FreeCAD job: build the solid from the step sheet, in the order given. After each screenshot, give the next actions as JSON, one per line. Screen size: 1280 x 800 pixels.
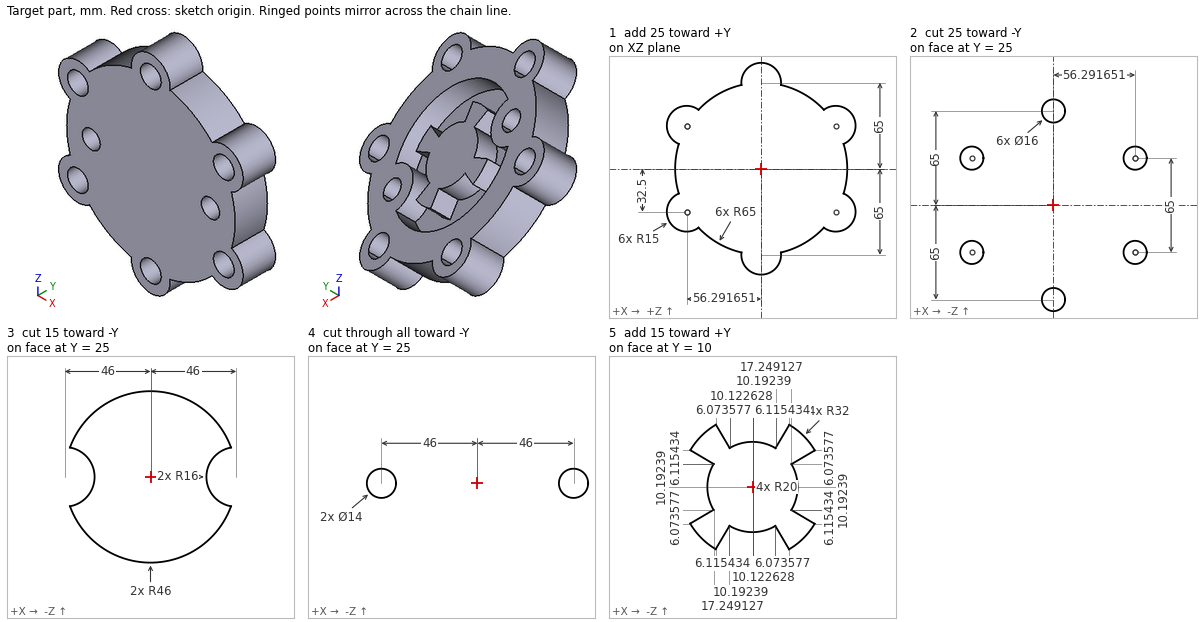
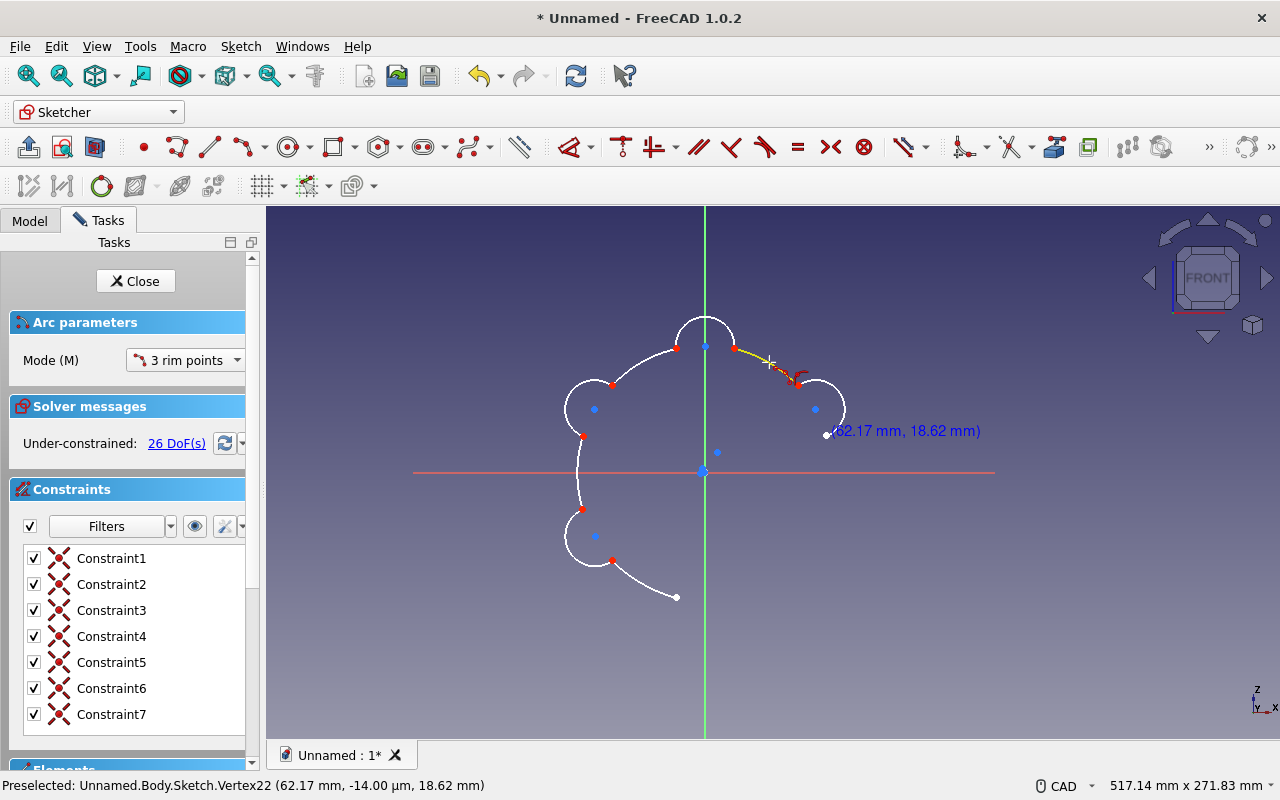
{"action": "left_click", "coordinate": [827, 509]}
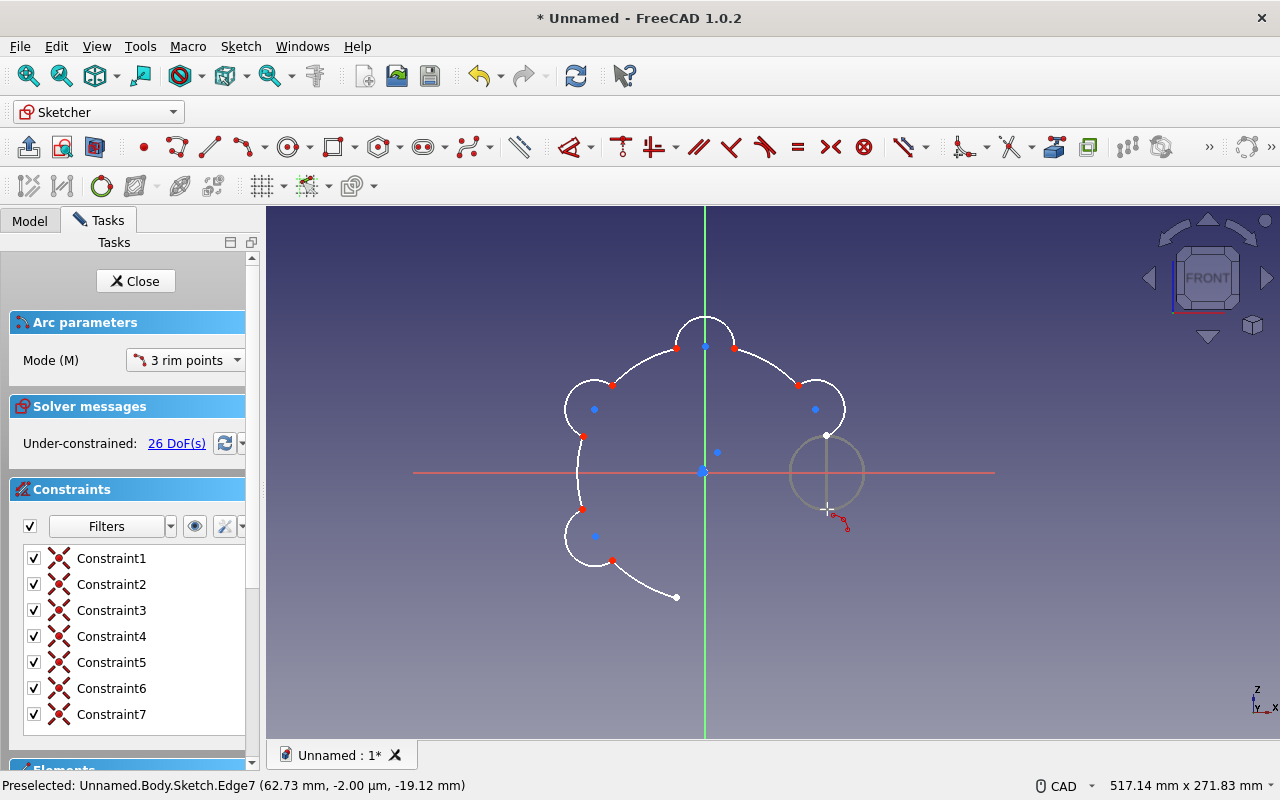
{"action": "scroll", "coordinate": [832, 480], "scroll_direction": "up", "scroll_amount": 6}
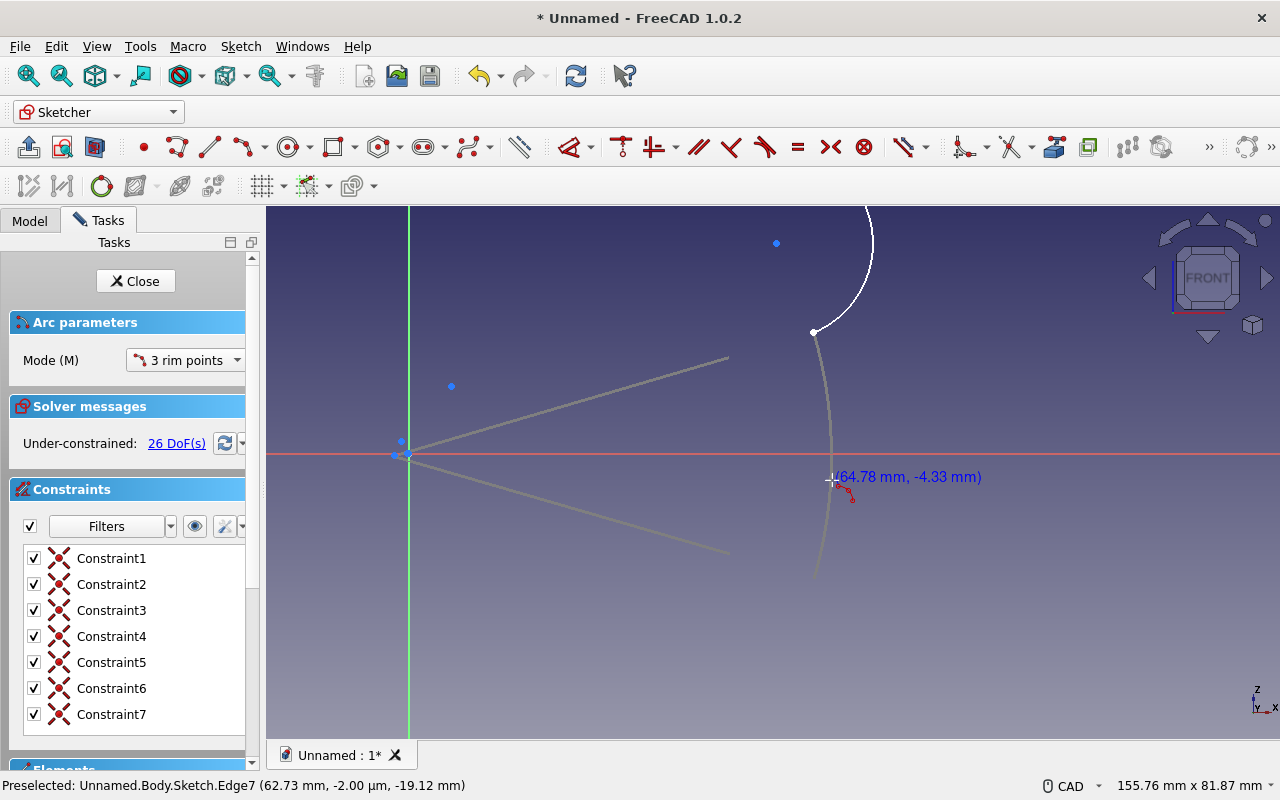
{"action": "left_click", "coordinate": [831, 479]}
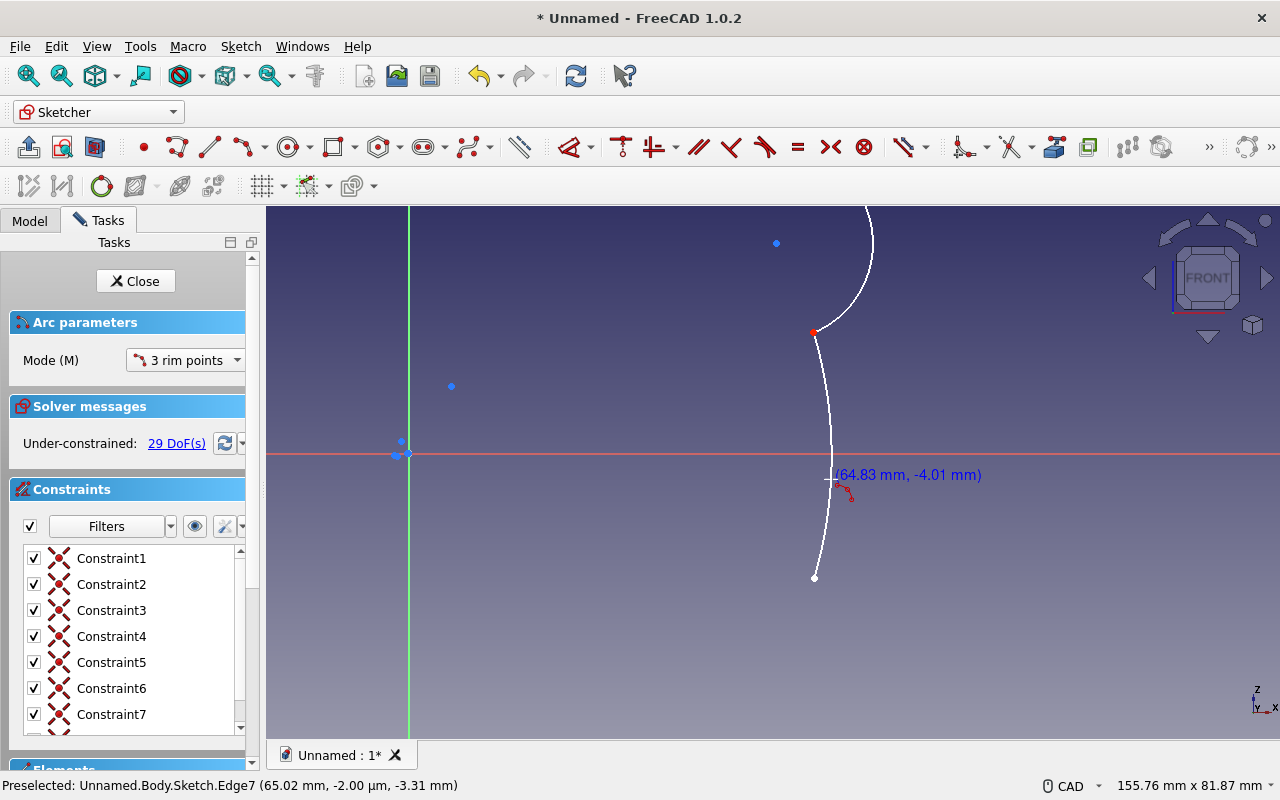
{"action": "left_click", "coordinate": [814, 578]}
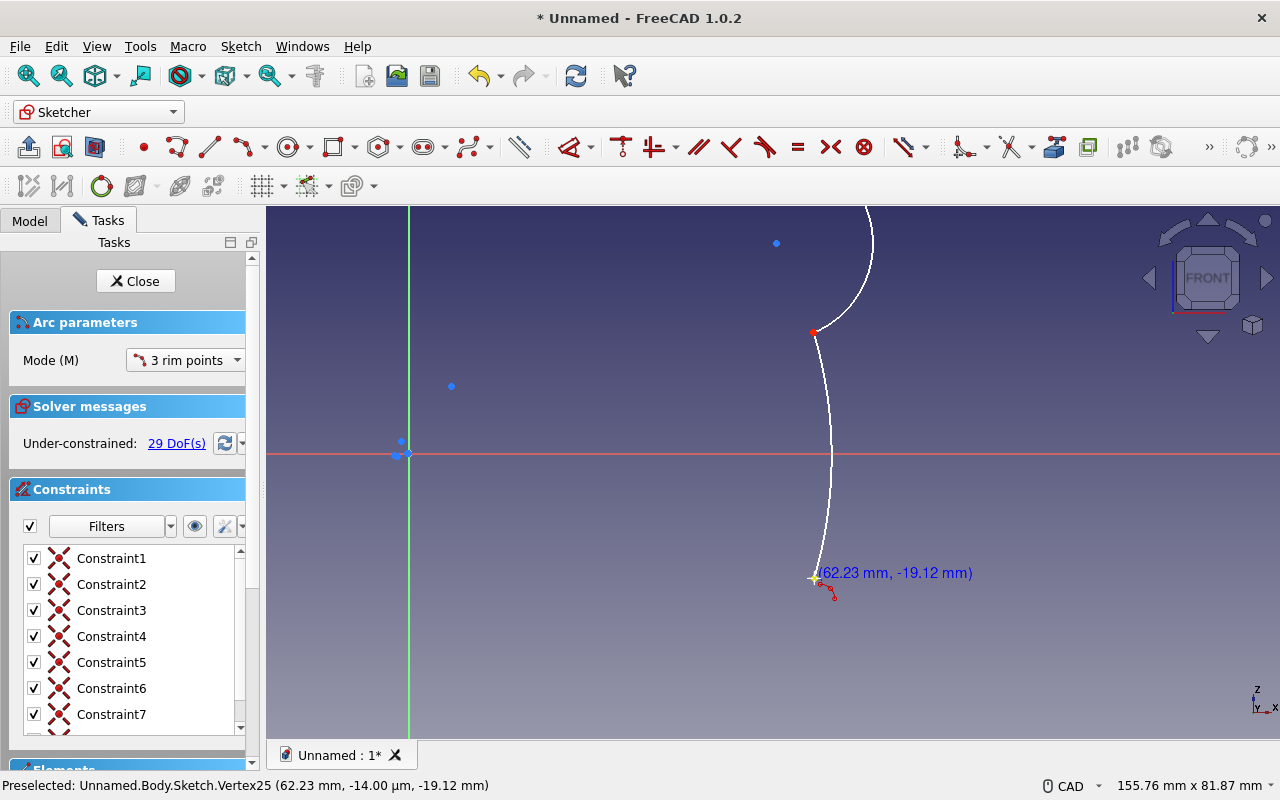
{"action": "scroll", "coordinate": [832, 481], "scroll_direction": "down", "scroll_amount": 6}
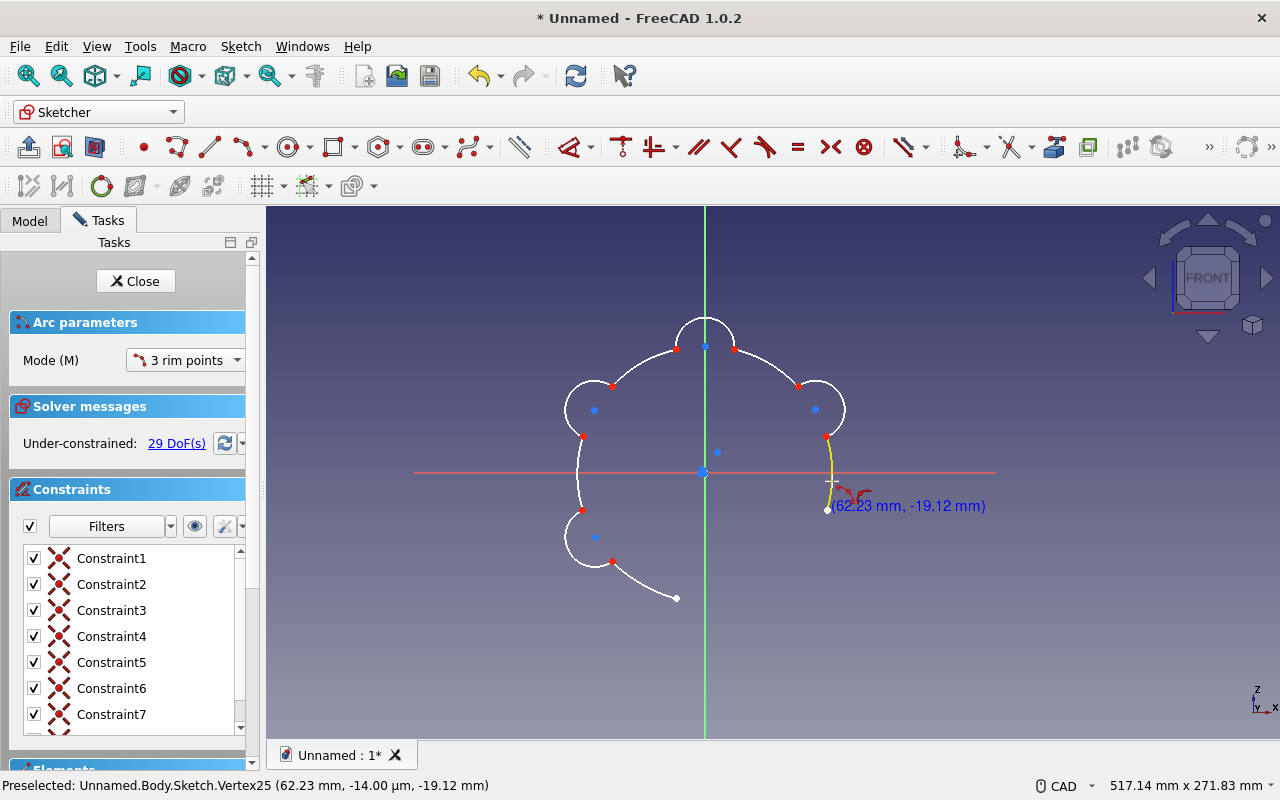
{"action": "left_click", "coordinate": [798, 561]}
{"action": "left_click", "coordinate": [841, 552]}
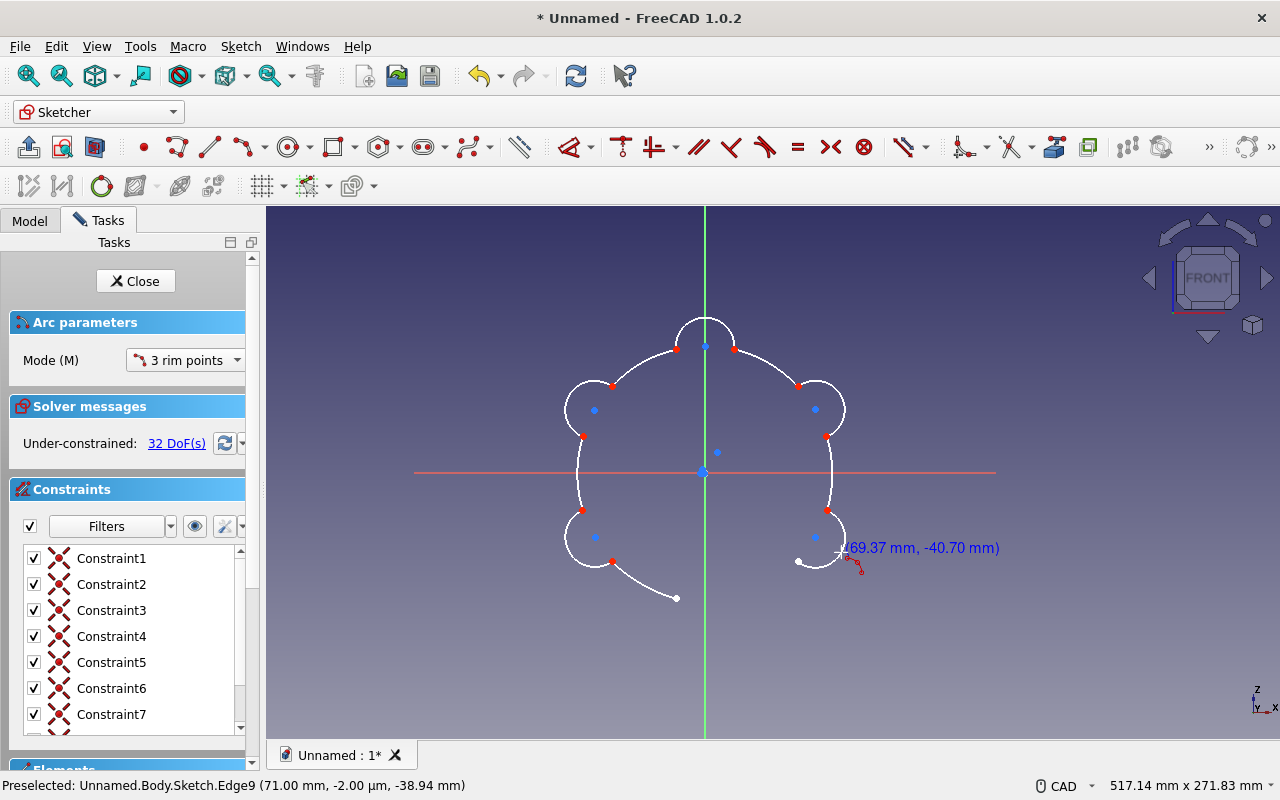
{"action": "left_click", "coordinate": [798, 562]}
{"action": "left_click", "coordinate": [734, 597]}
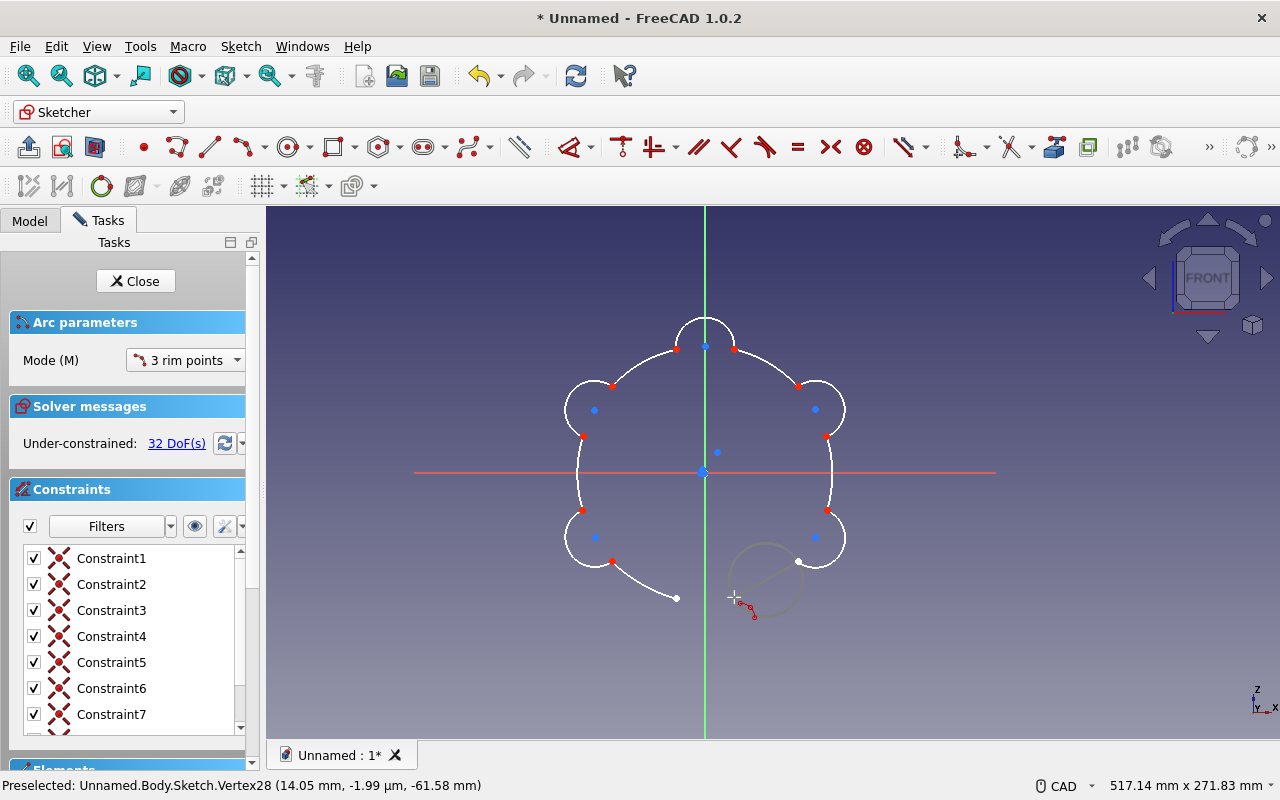
{"action": "scroll", "coordinate": [769, 584], "scroll_direction": "up", "scroll_amount": 6}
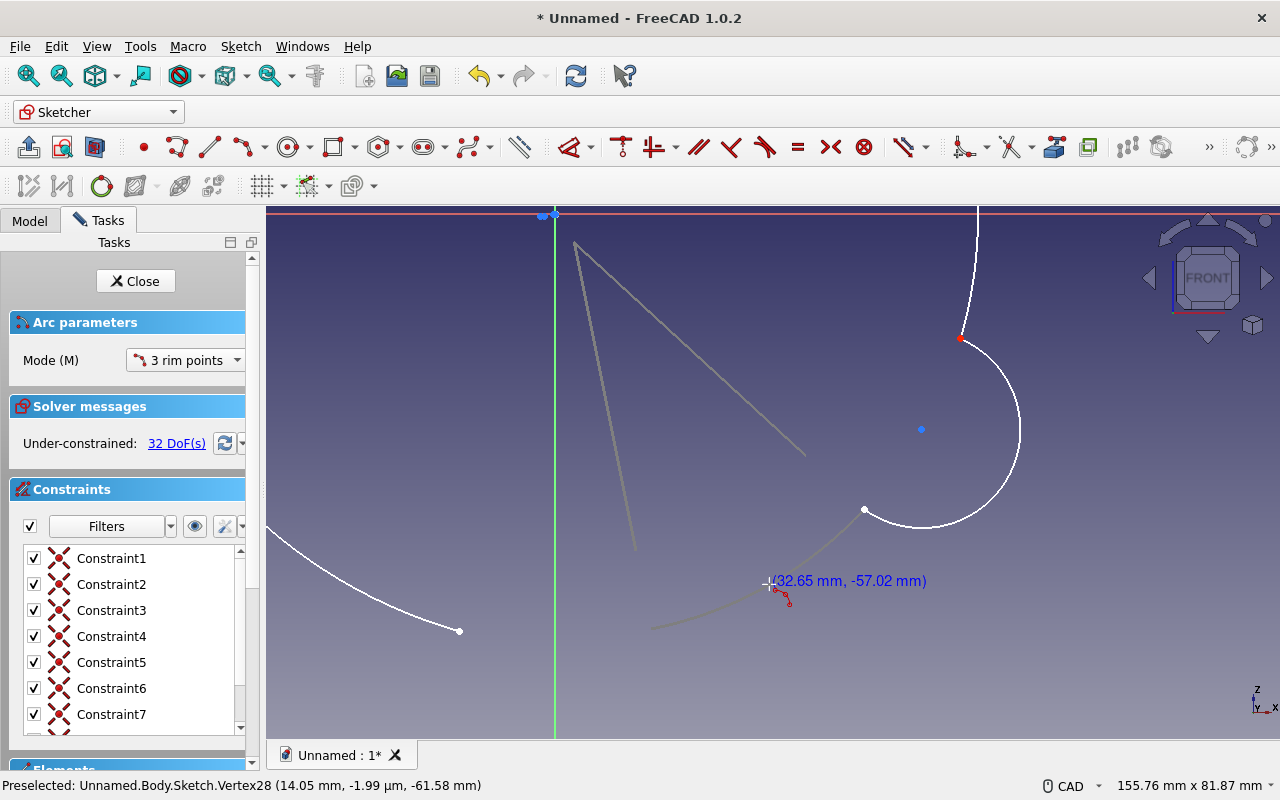
{"action": "left_click", "coordinate": [767, 581]}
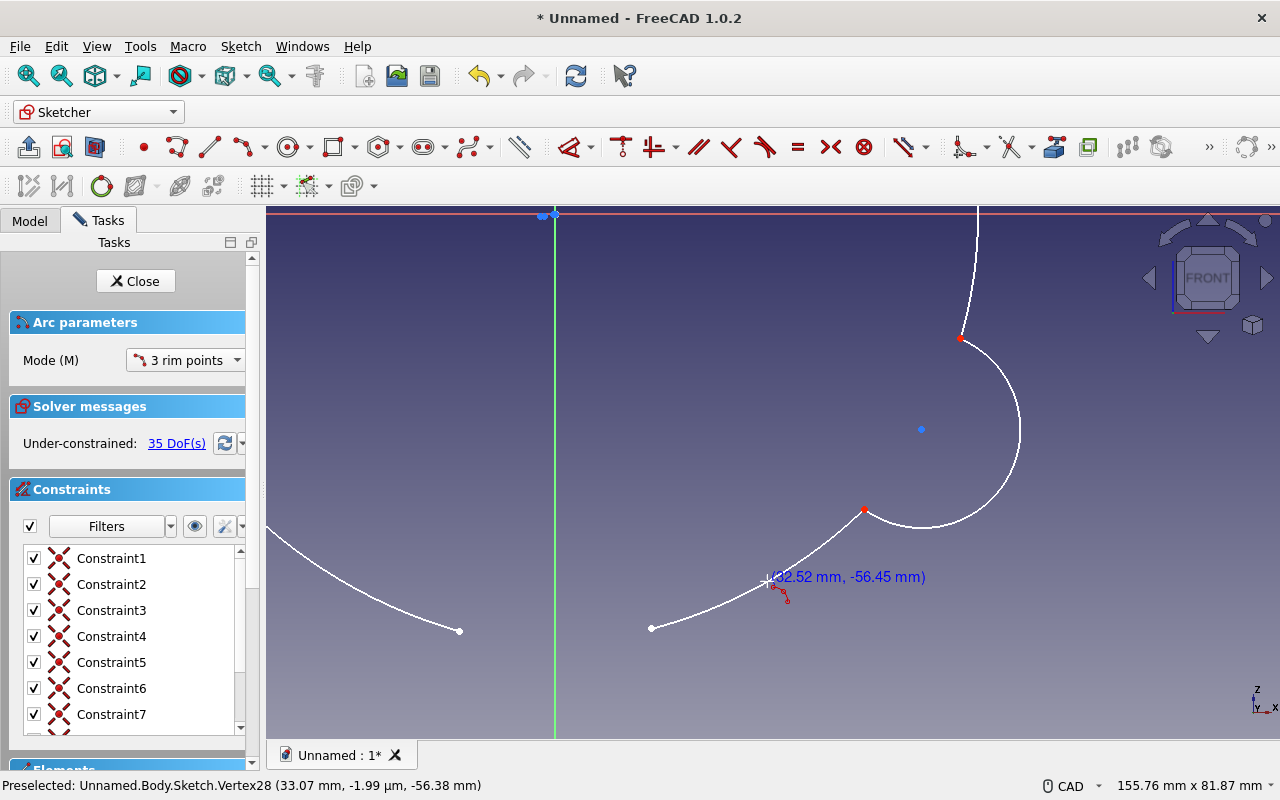
{"action": "left_click", "coordinate": [652, 629]}
{"action": "left_click", "coordinate": [459, 631]}